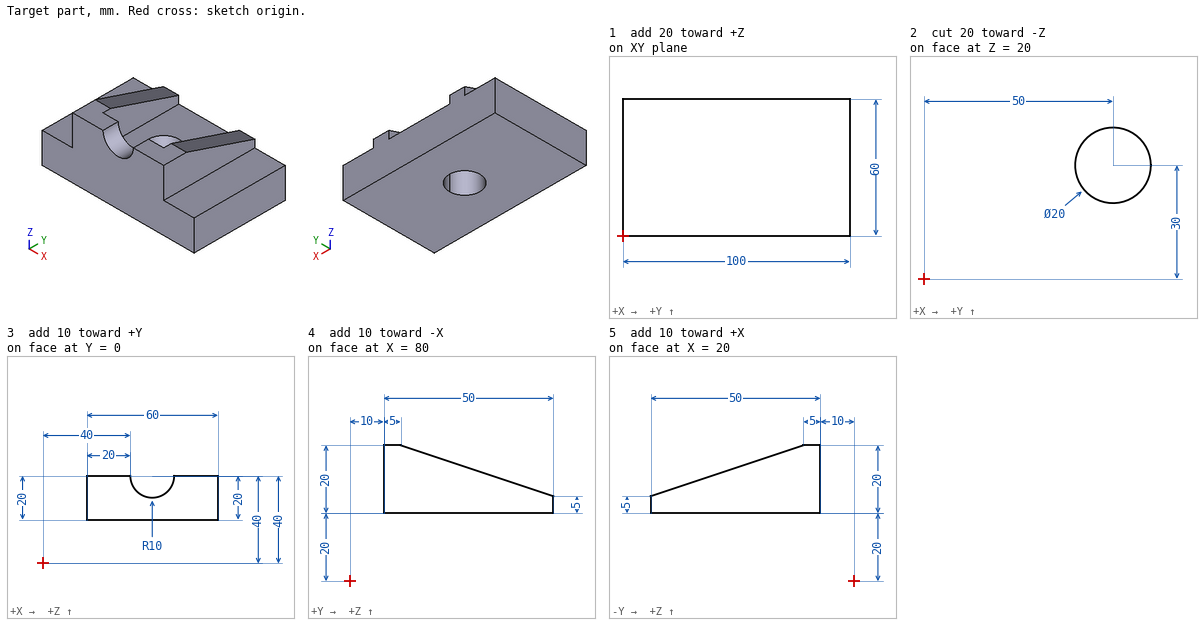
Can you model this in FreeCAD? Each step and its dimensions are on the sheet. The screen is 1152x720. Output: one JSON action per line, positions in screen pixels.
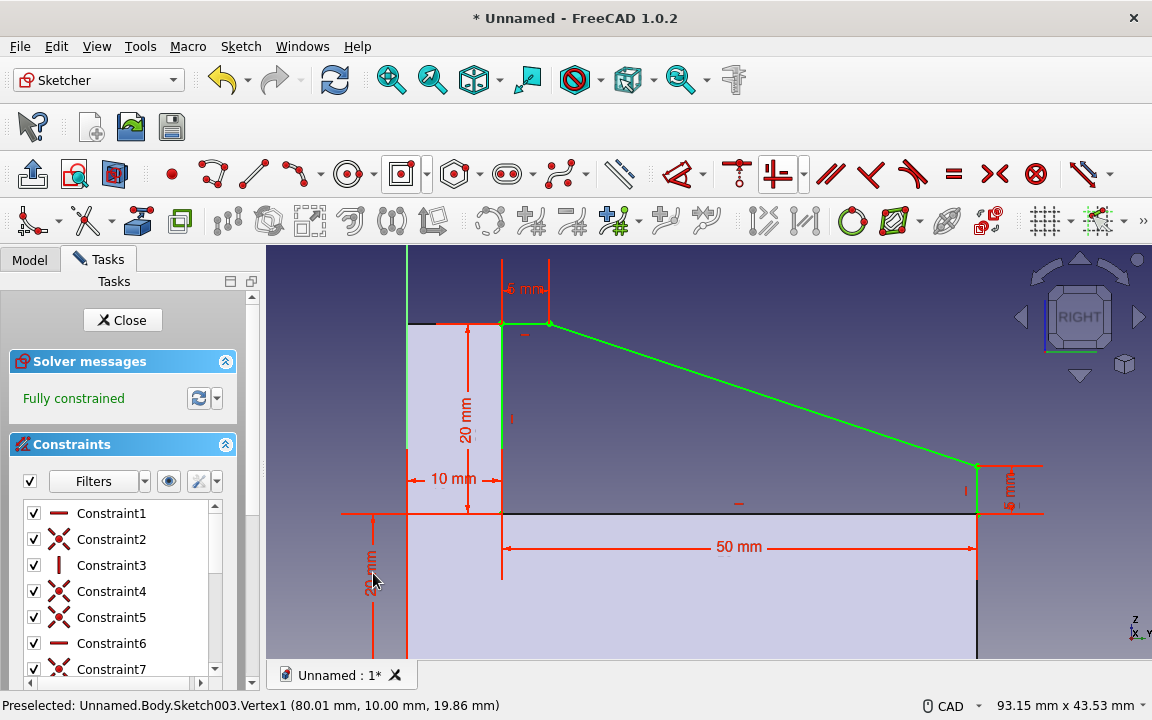
{"action": "left_click", "coordinate": [123, 320]}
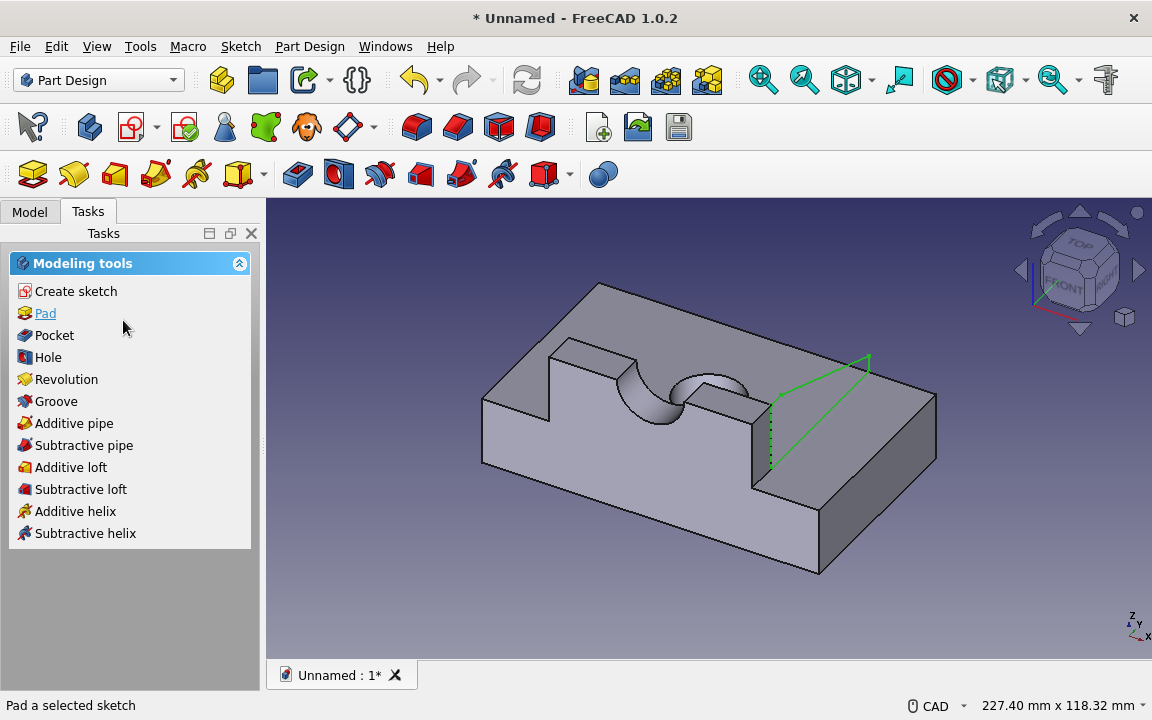
{"action": "left_click", "coordinate": [33, 174]}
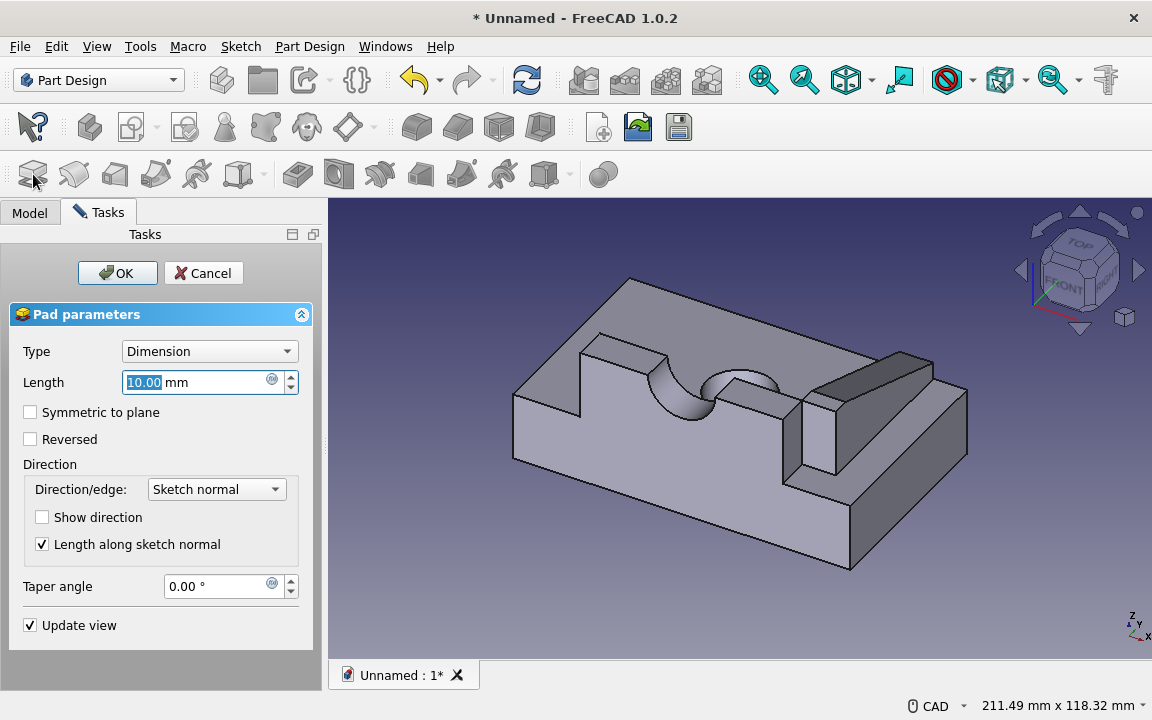
{"action": "type", "text": "10"}
{"action": "key", "text": "Tab"}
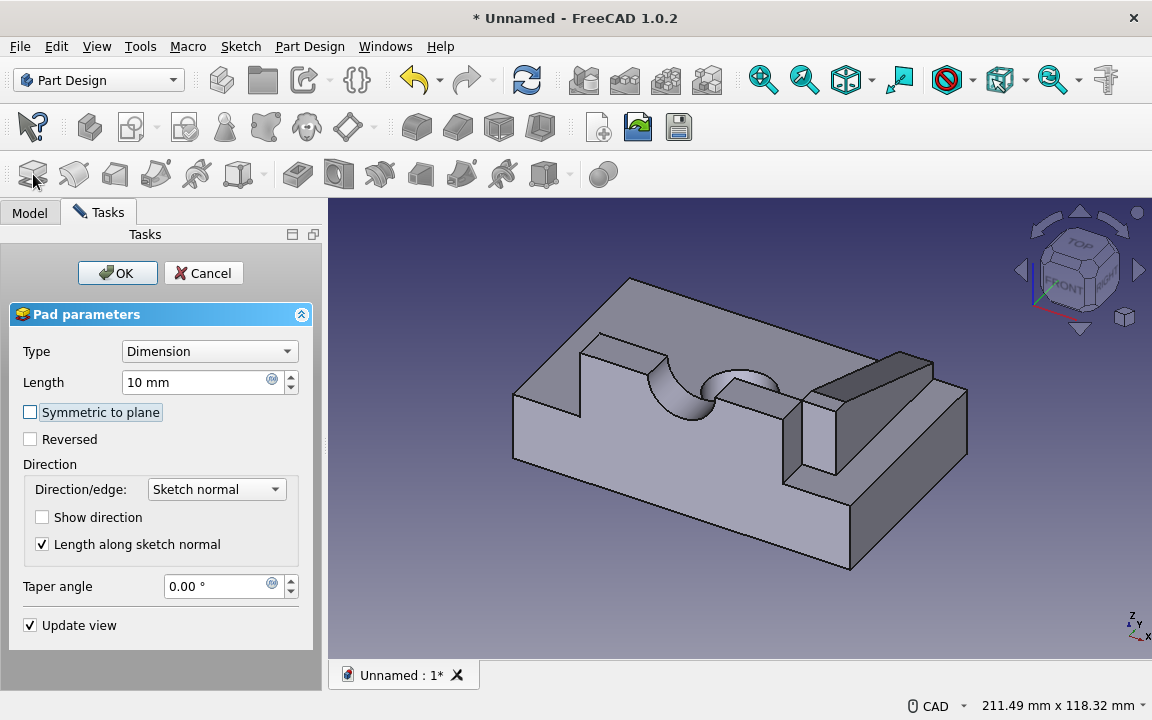
{"action": "left_click", "coordinate": [31, 439]}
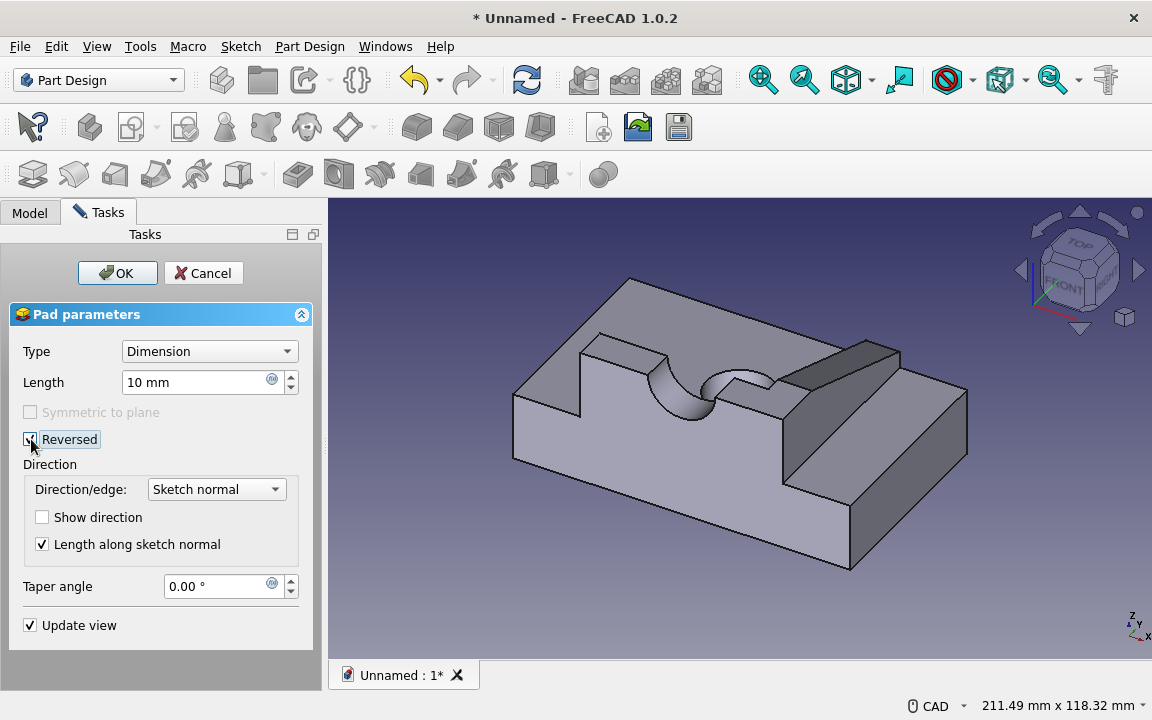
{"action": "left_click", "coordinate": [118, 273]}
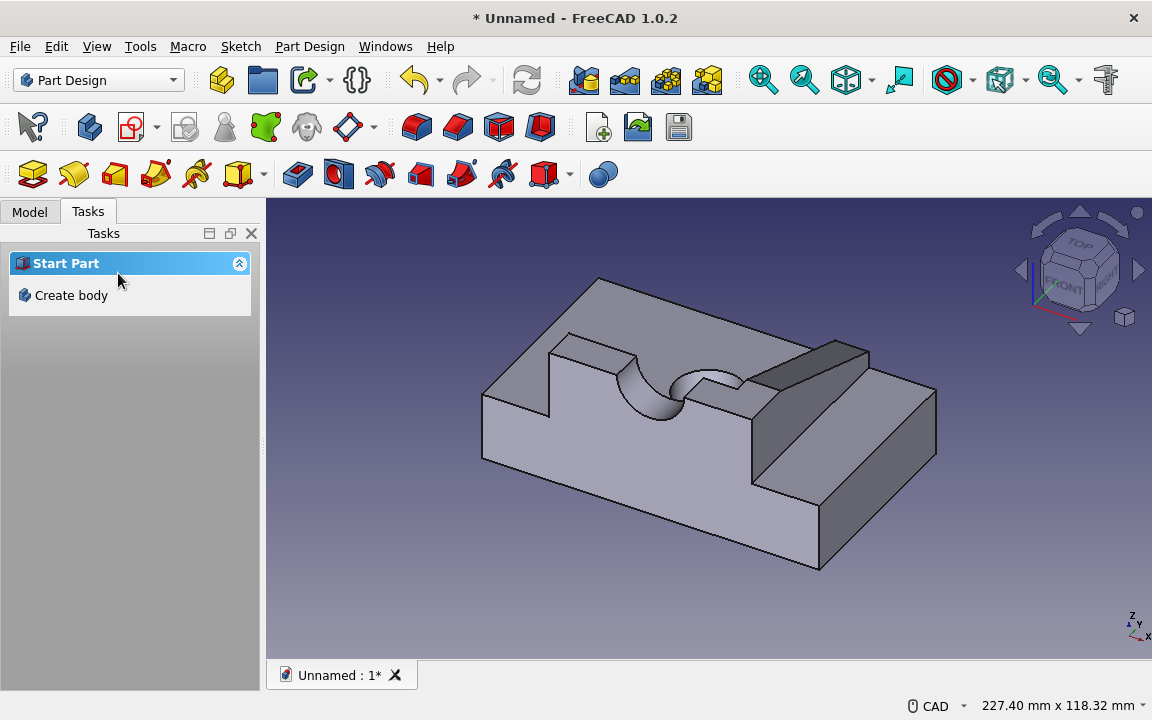
{"action": "key", "text": "6"}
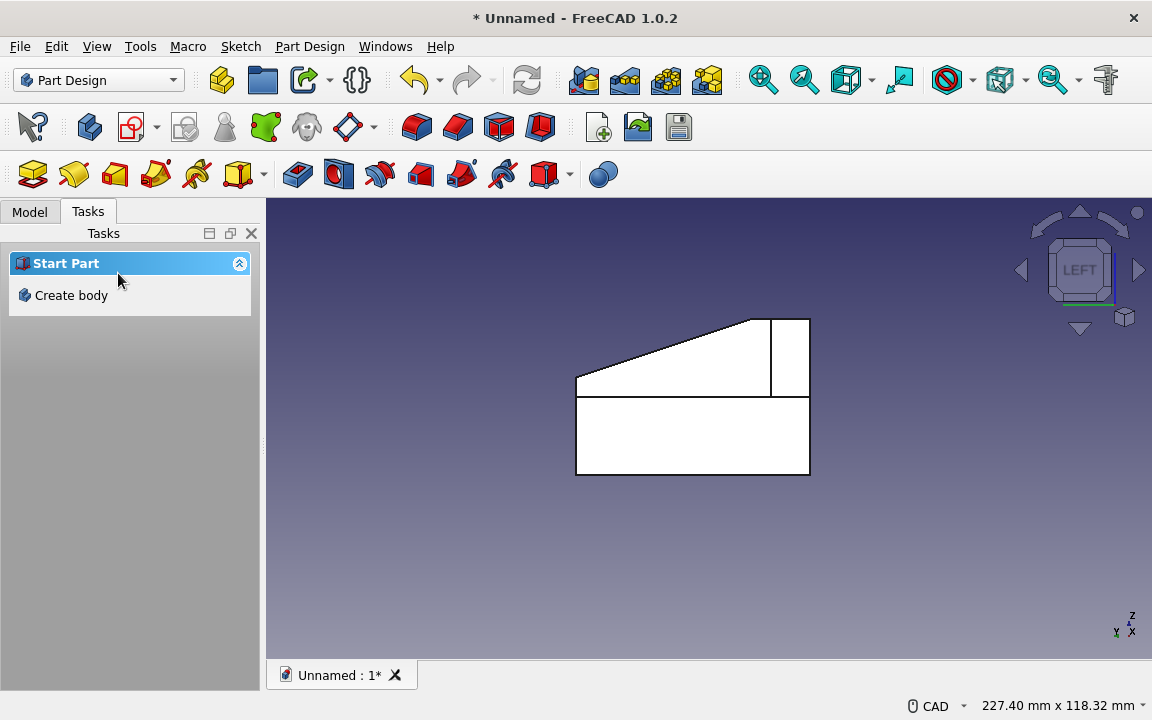
{"action": "left_click", "coordinate": [764, 80]}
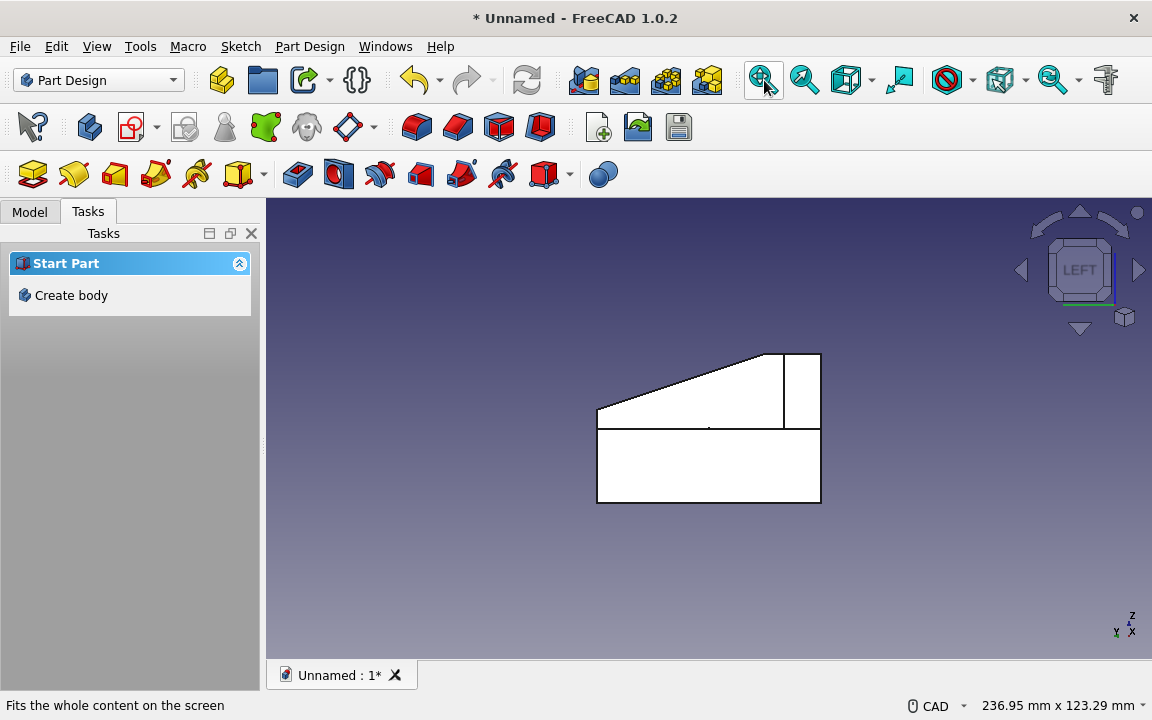
{"action": "left_click", "coordinate": [802, 379]}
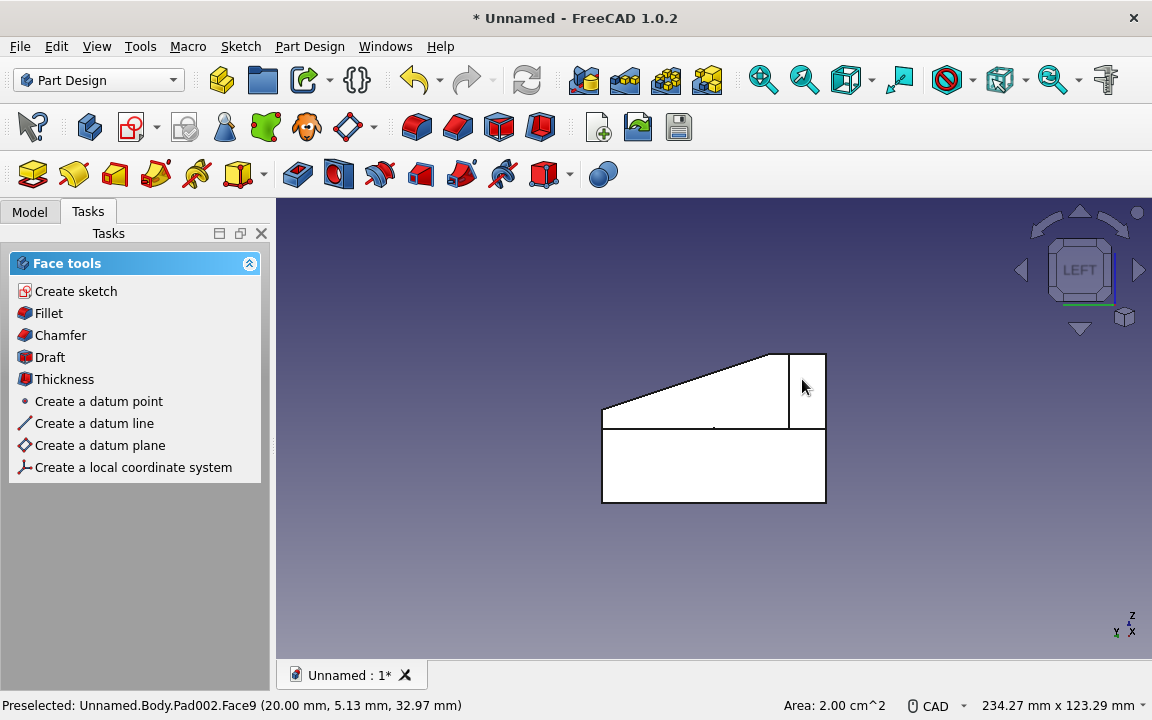
{"action": "left_click", "coordinate": [130, 128]}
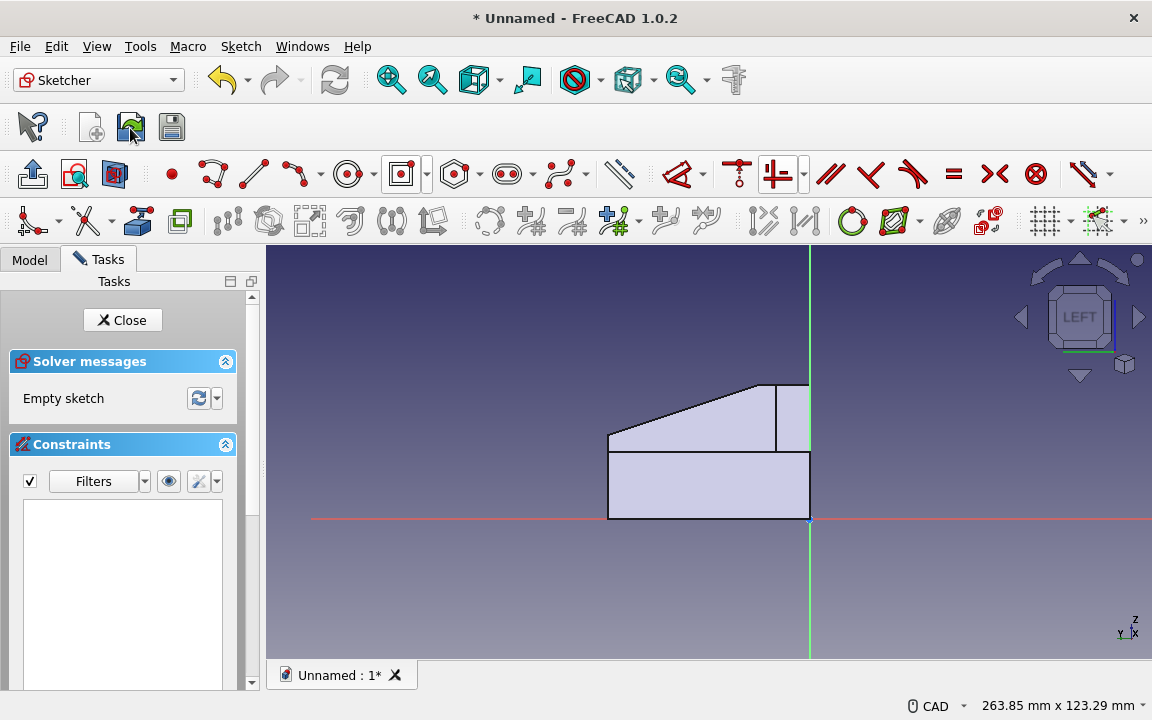
{"action": "scroll", "coordinate": [792, 452], "scroll_direction": "up", "scroll_amount": 3}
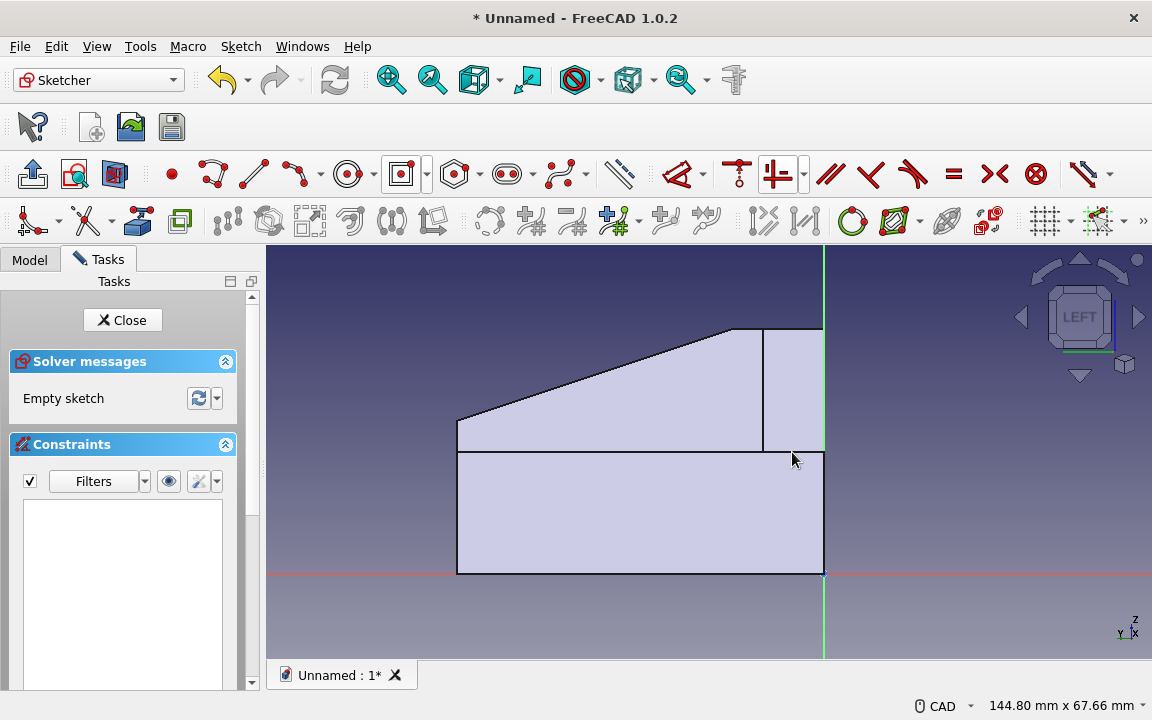
{"action": "left_click", "coordinate": [213, 174]}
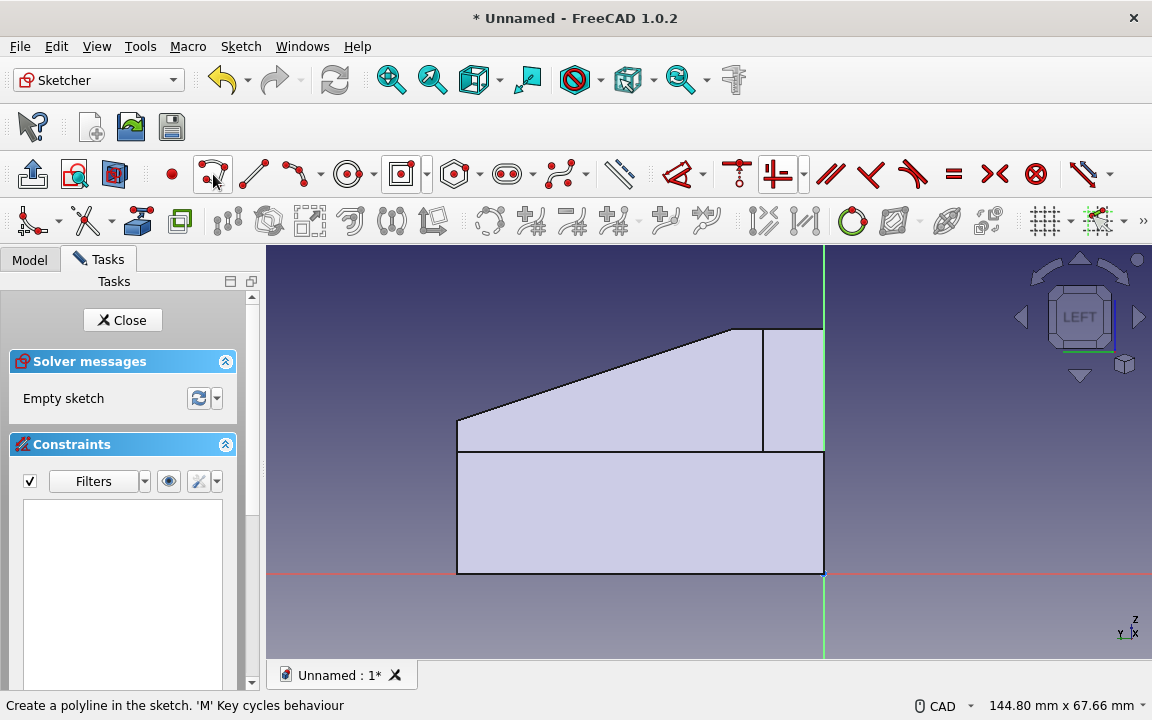
{"action": "left_click", "coordinate": [763, 452]}
{"action": "left_click", "coordinate": [763, 329]}
{"action": "left_click", "coordinate": [732, 329]}
{"action": "left_click", "coordinate": [457, 421]}
{"action": "left_click", "coordinate": [457, 452]}
{"action": "left_click", "coordinate": [763, 453]}
{"action": "key", "text": "Escape"}
{"action": "key", "text": "Escape"}